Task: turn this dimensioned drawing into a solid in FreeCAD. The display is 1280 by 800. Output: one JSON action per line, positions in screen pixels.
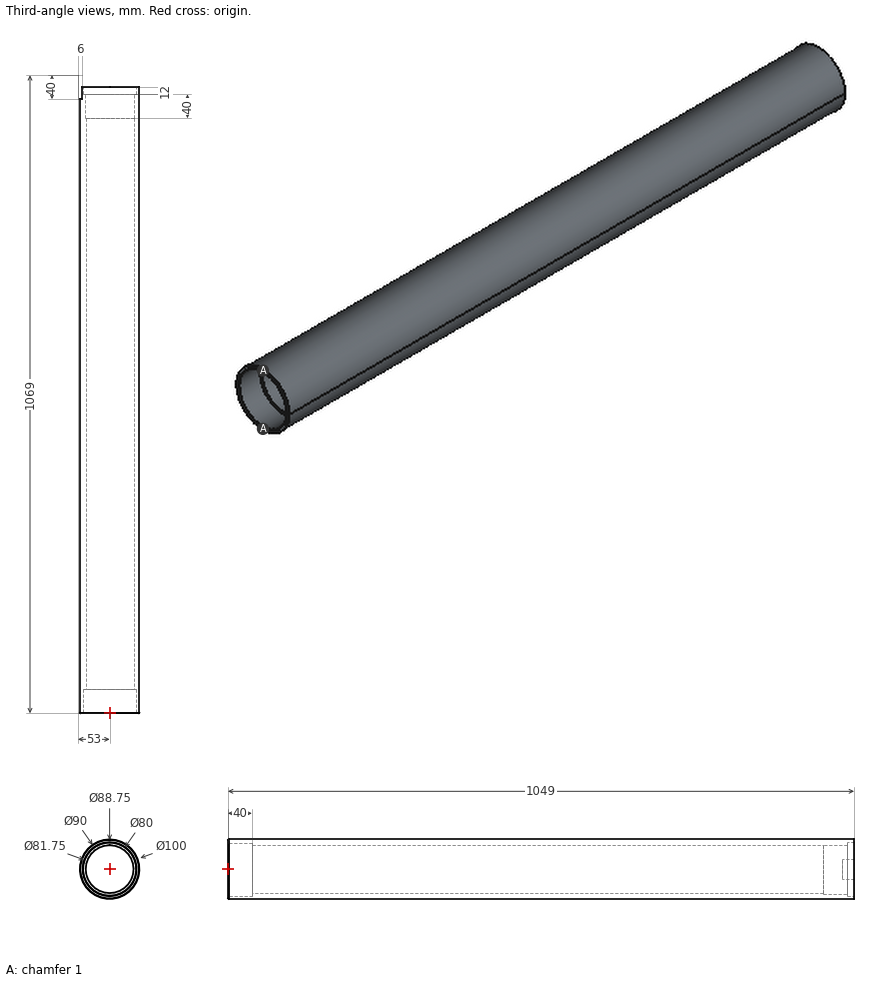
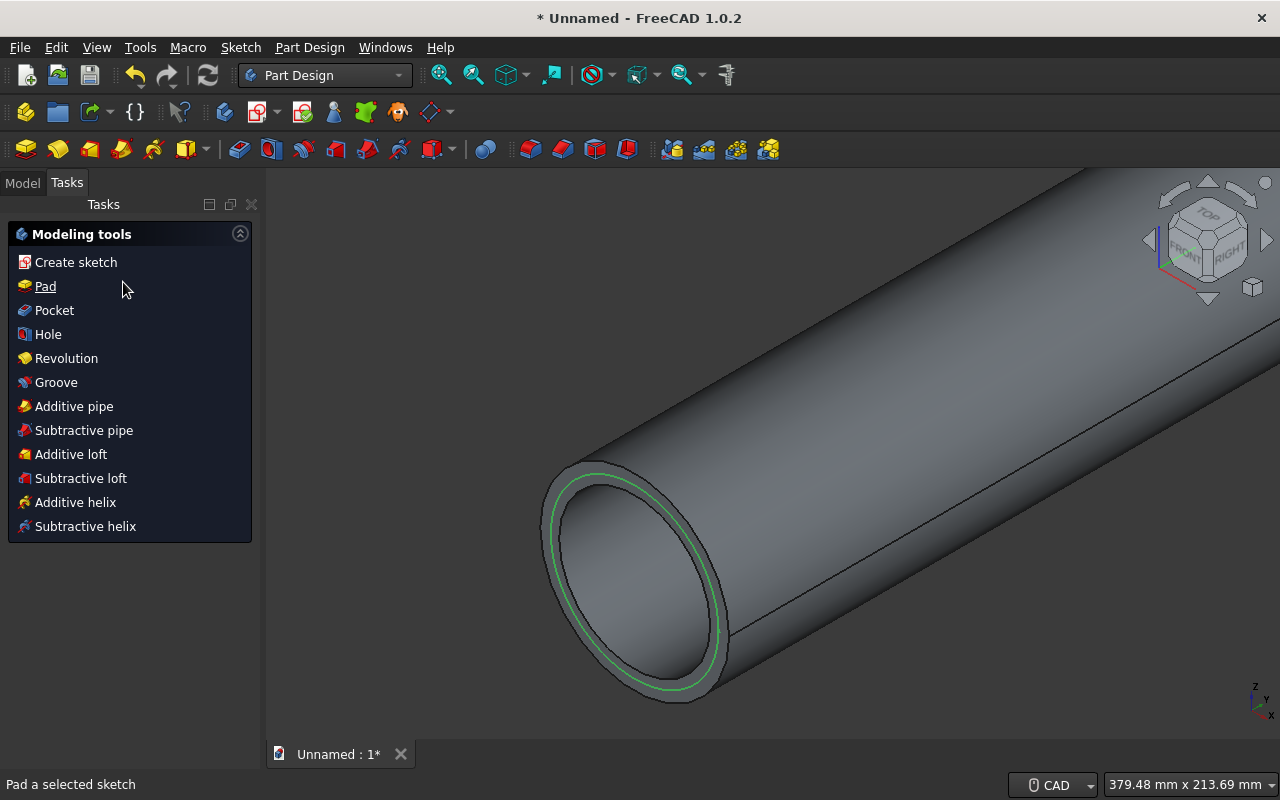
{"action": "left_click", "coordinate": [240, 150]}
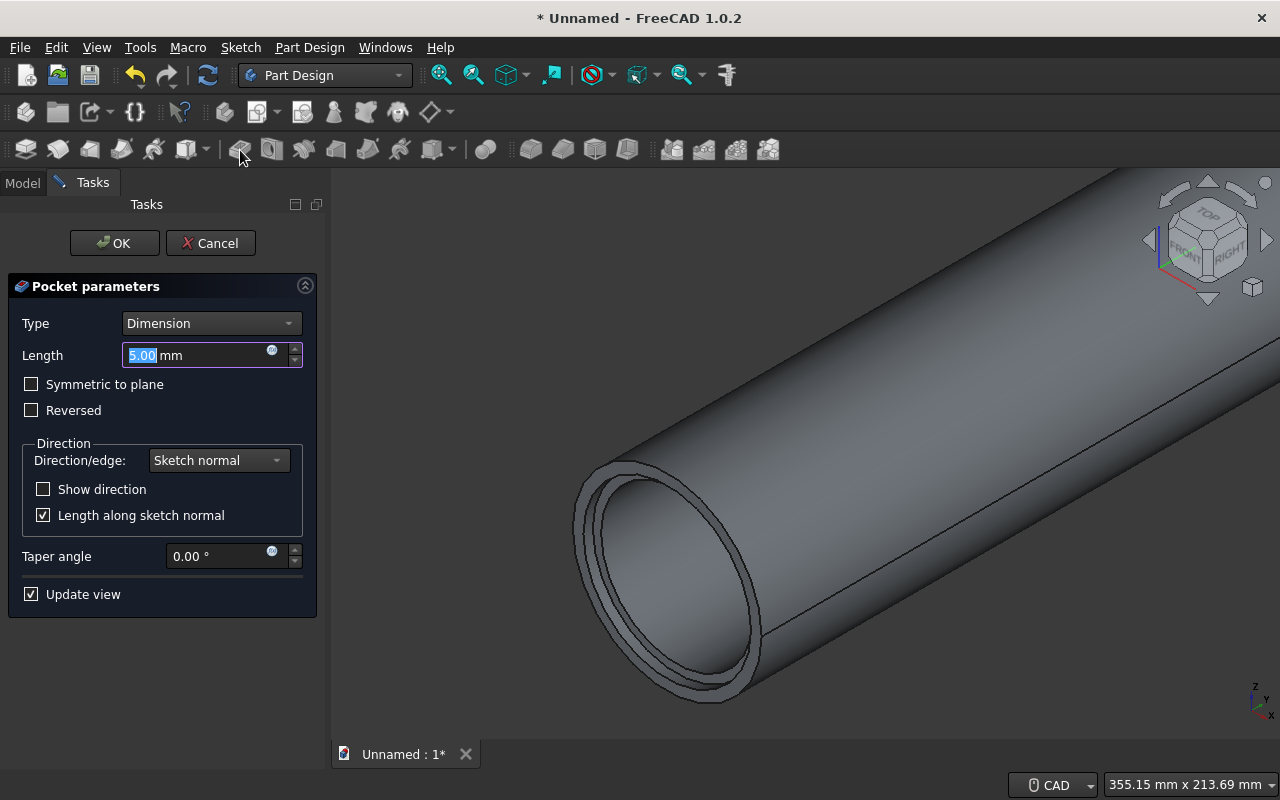
{"action": "type", "text": "40"}
{"action": "key", "text": "Tab"}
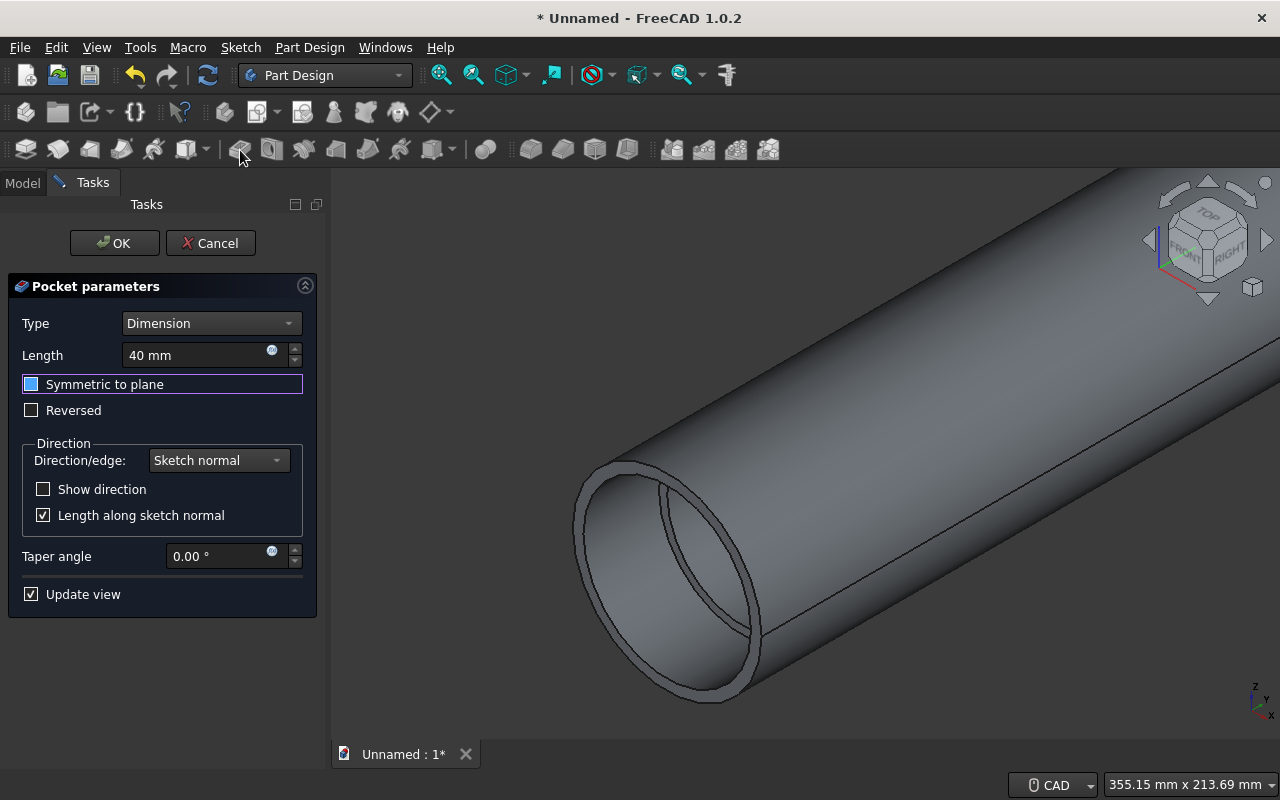
{"action": "left_click", "coordinate": [115, 243]}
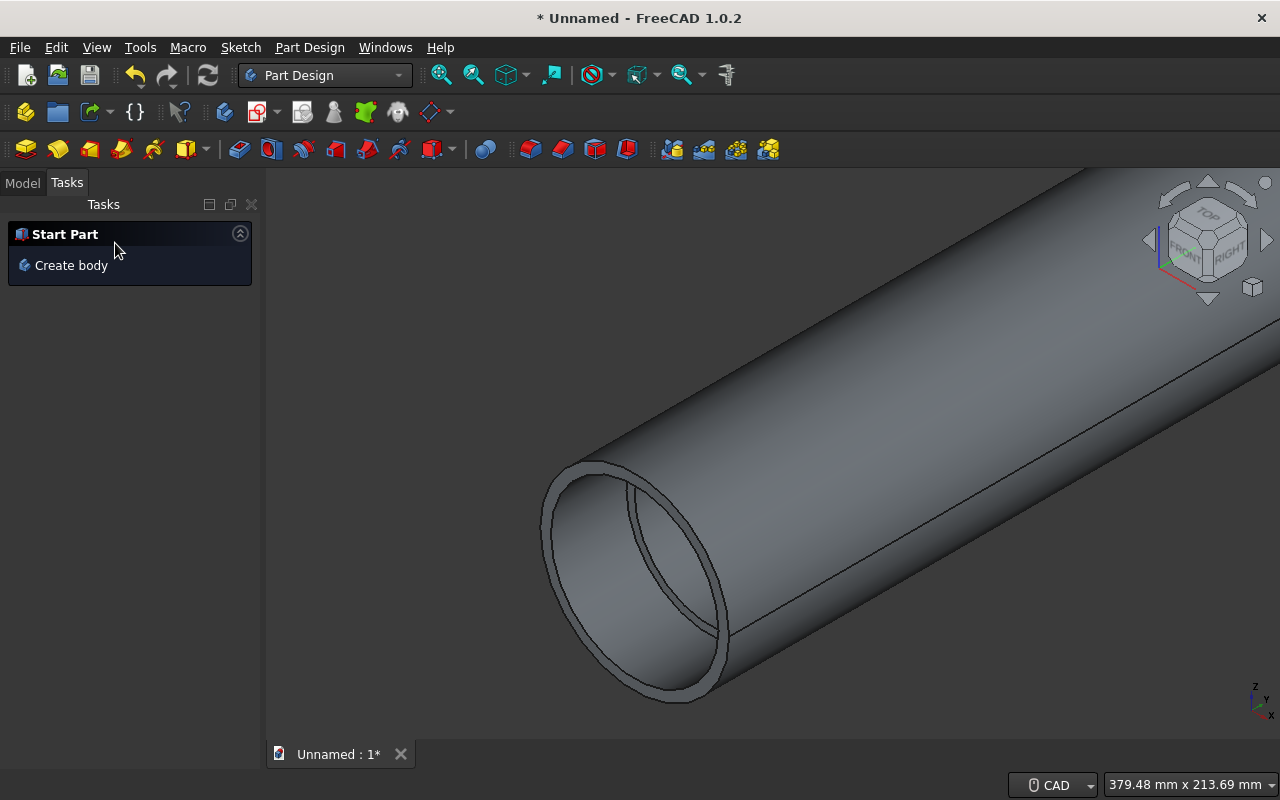
{"action": "left_click", "coordinate": [442, 76]}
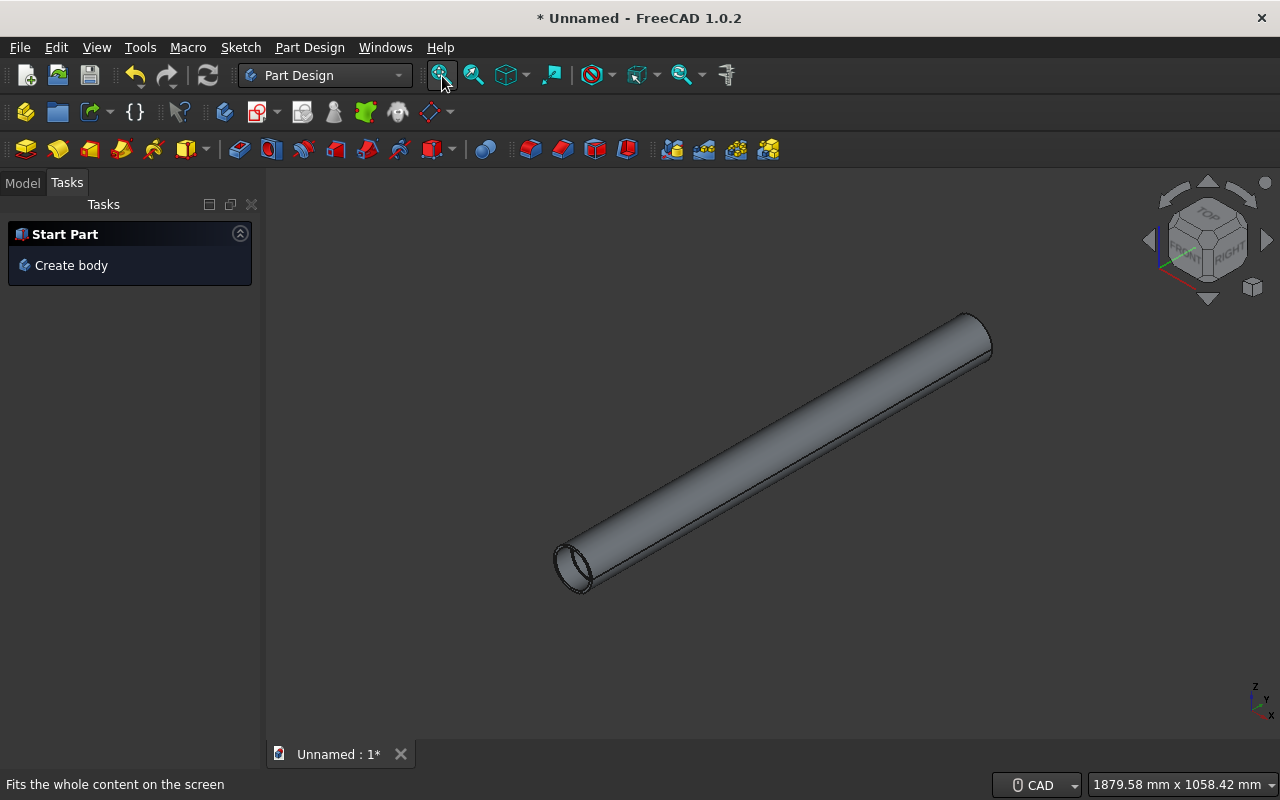
{"action": "left_click", "coordinate": [556, 558]}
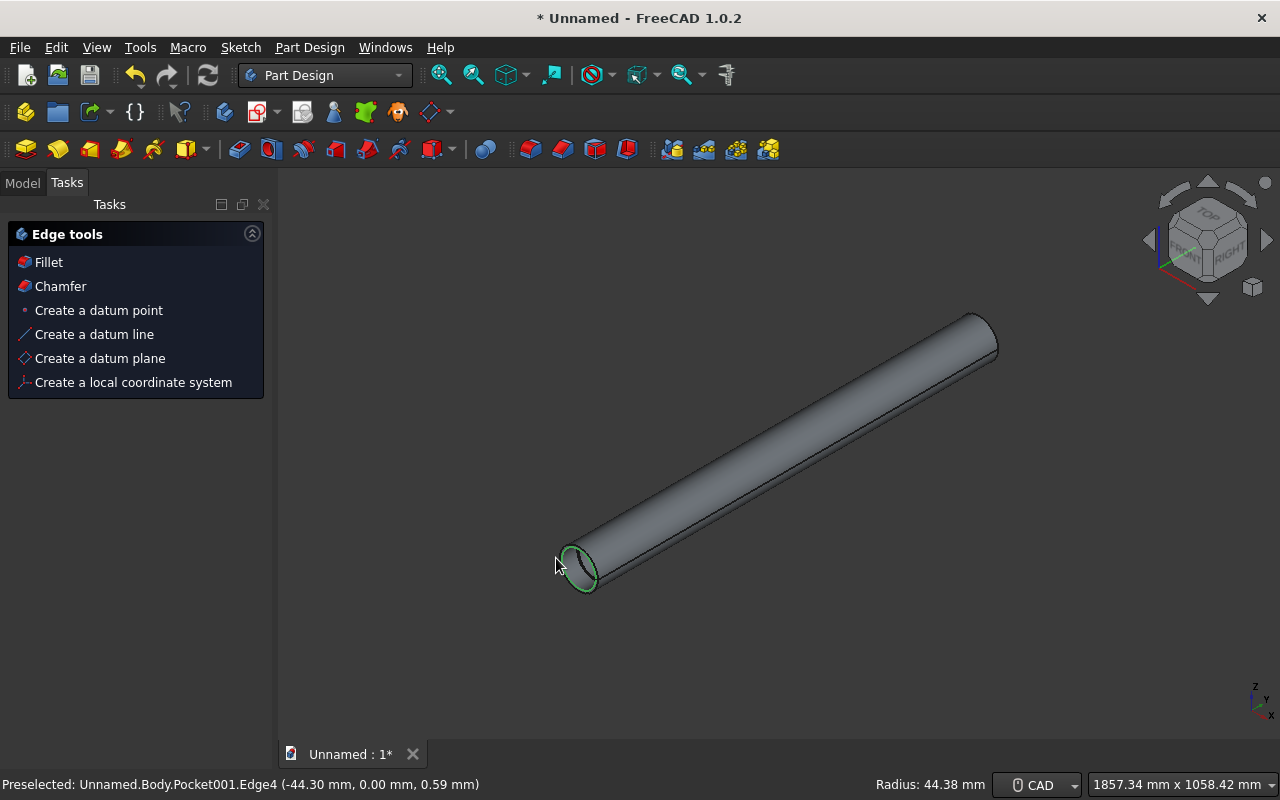
{"action": "left_click", "coordinate": [573, 544], "text": "ctrl"}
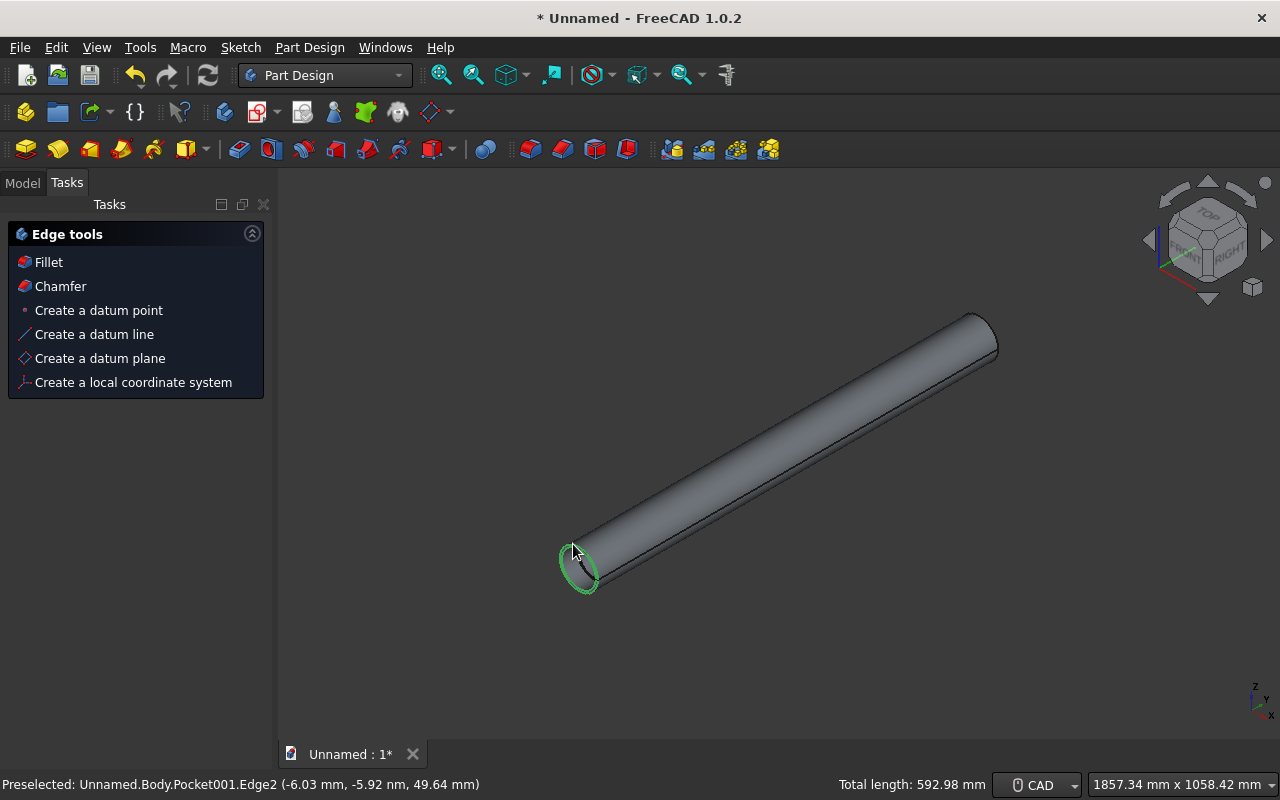
{"action": "left_click", "coordinate": [564, 150]}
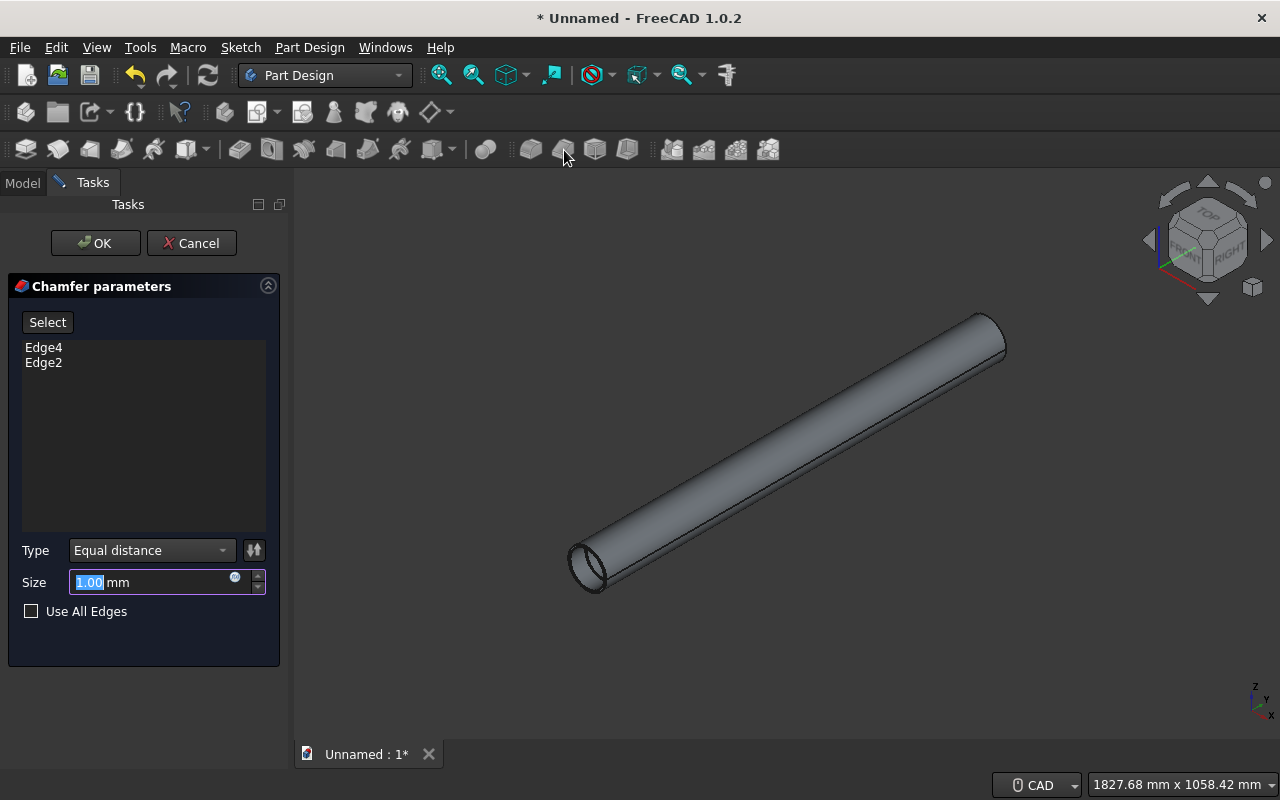
{"action": "type", "text": "1"}
{"action": "key", "text": "Tab"}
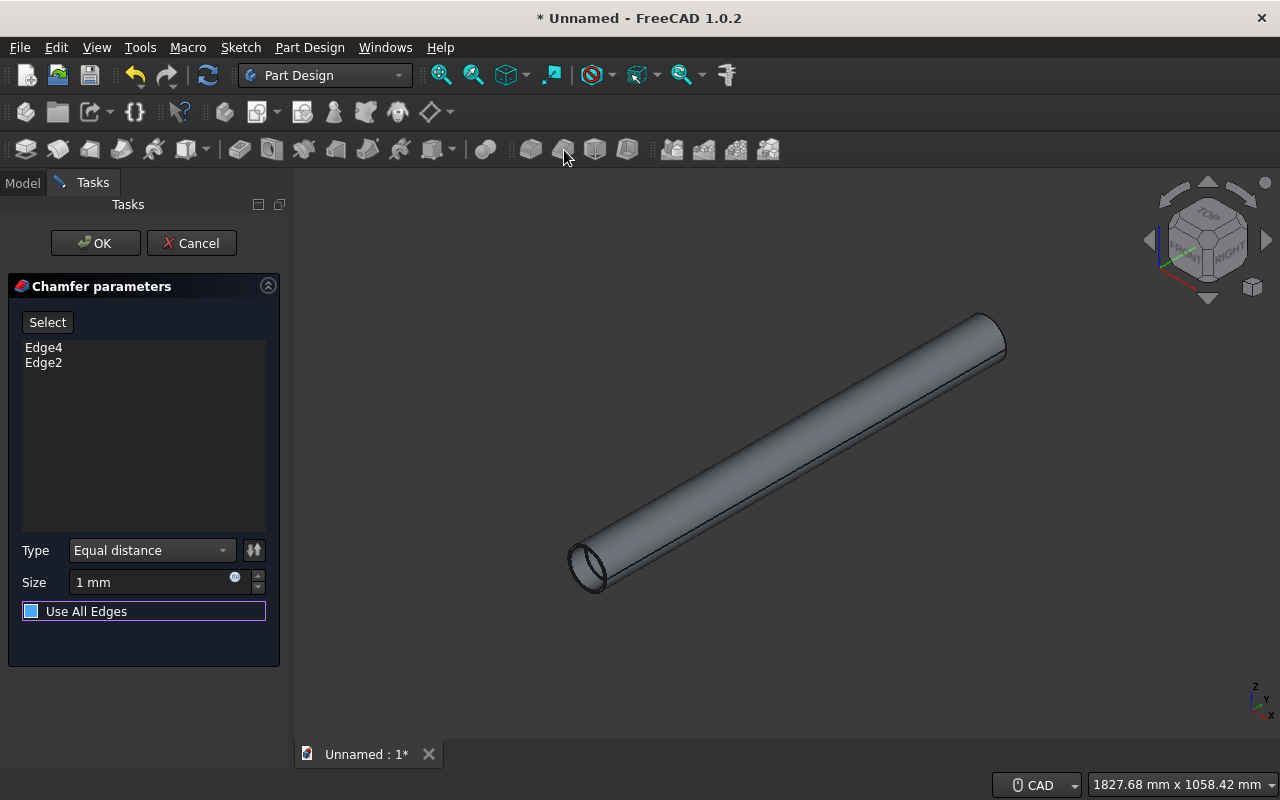
{"action": "left_click", "coordinate": [96, 243]}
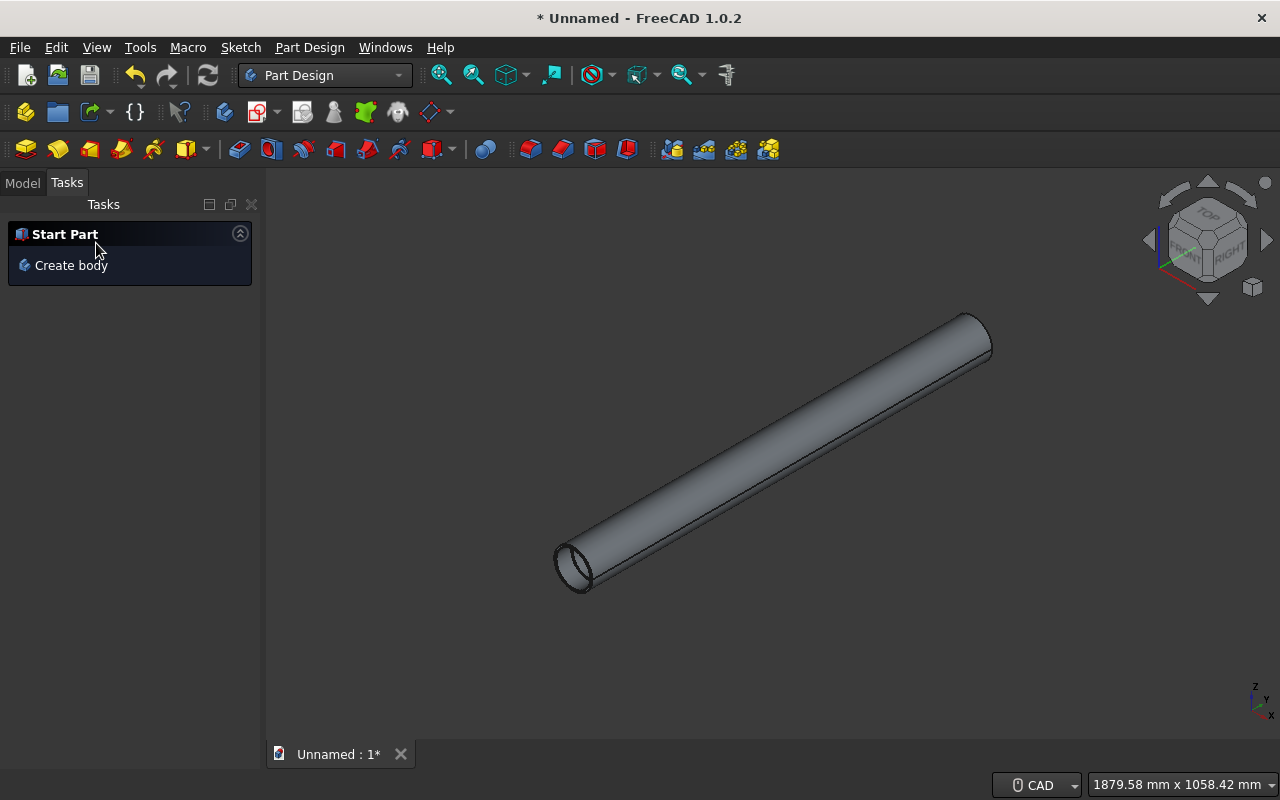
{"action": "key", "text": "4"}